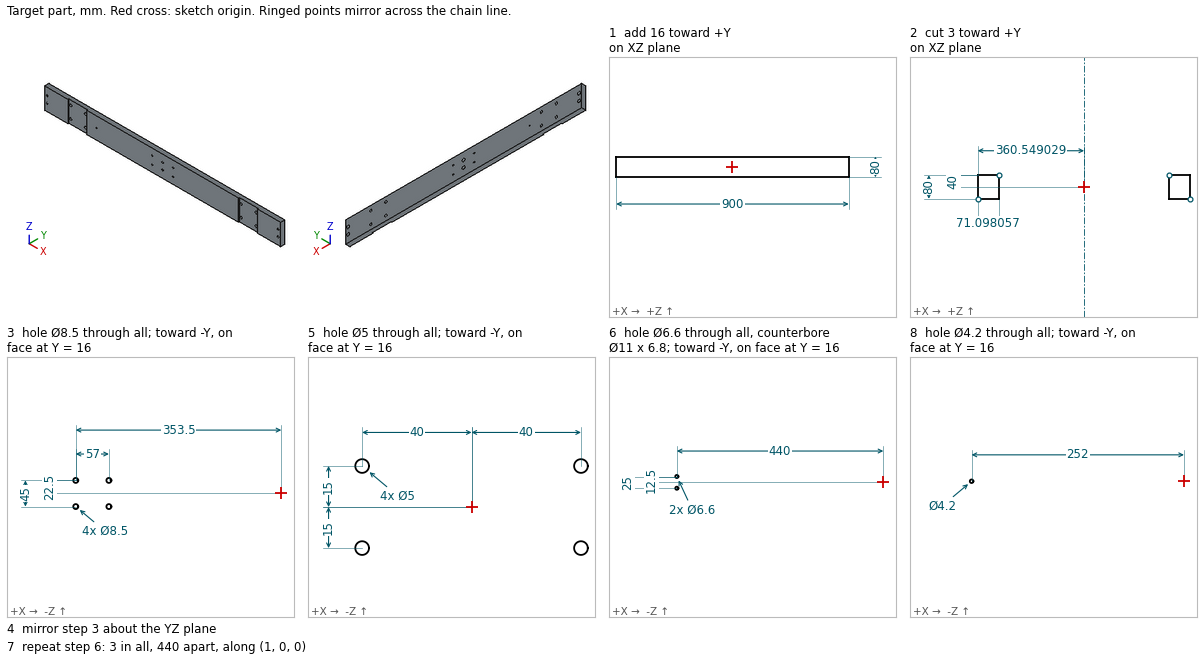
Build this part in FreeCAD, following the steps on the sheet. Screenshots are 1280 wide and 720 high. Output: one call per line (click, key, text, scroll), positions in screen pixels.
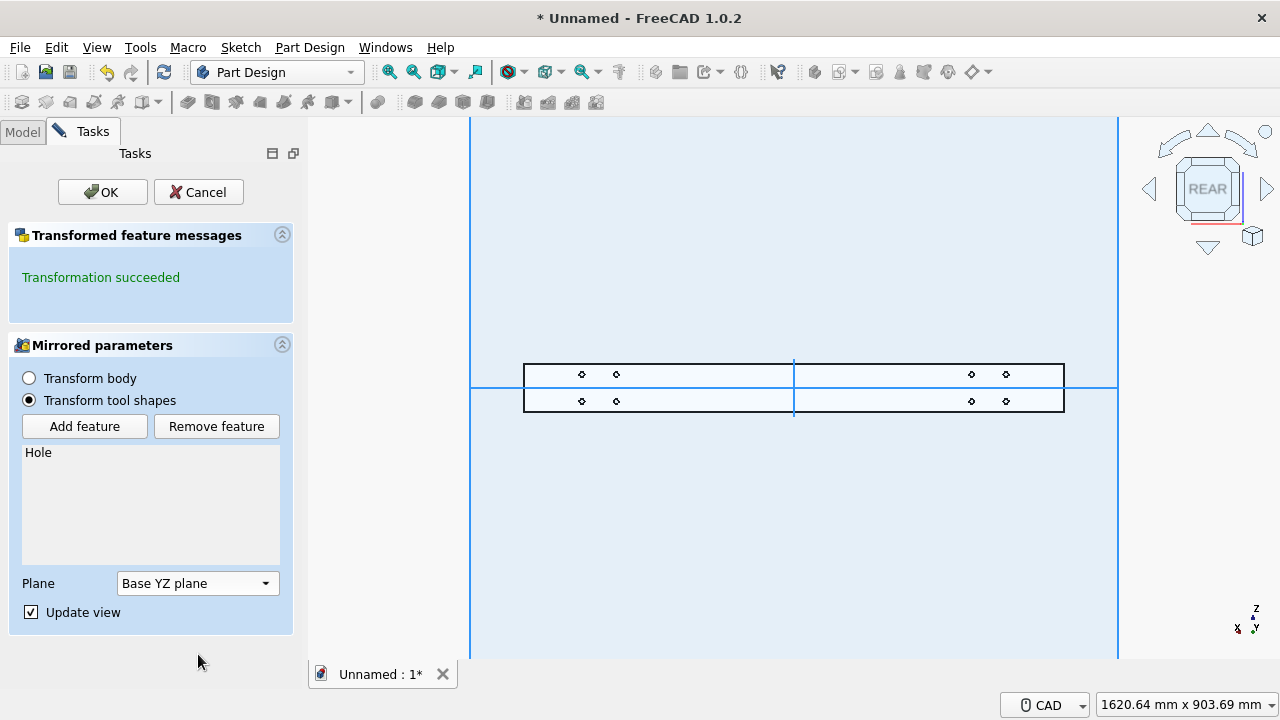
click(103, 192)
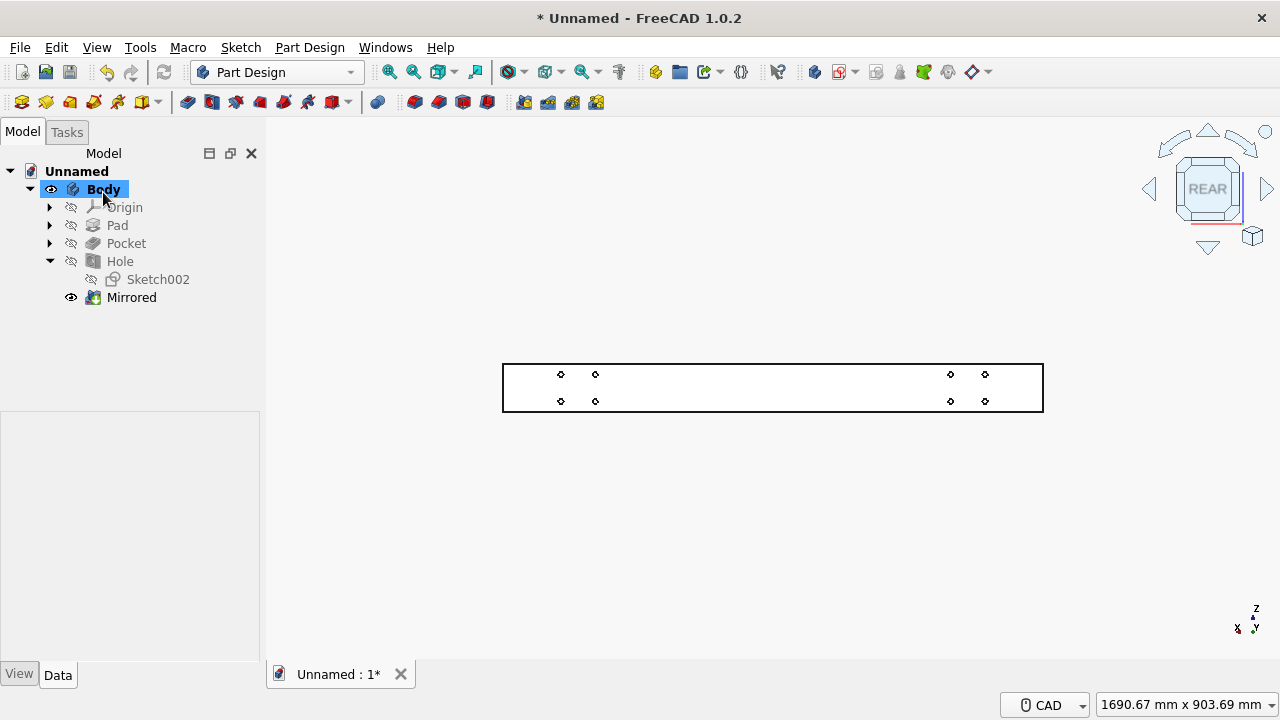
click(619, 387)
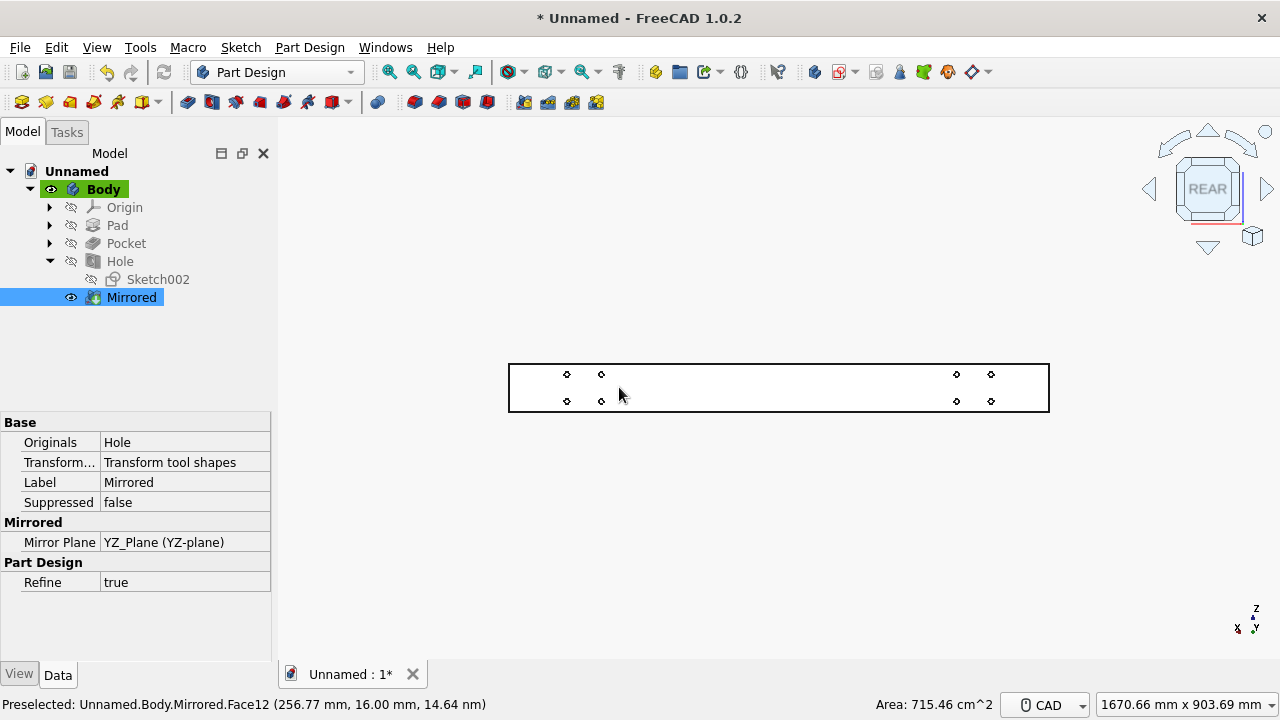
click(840, 72)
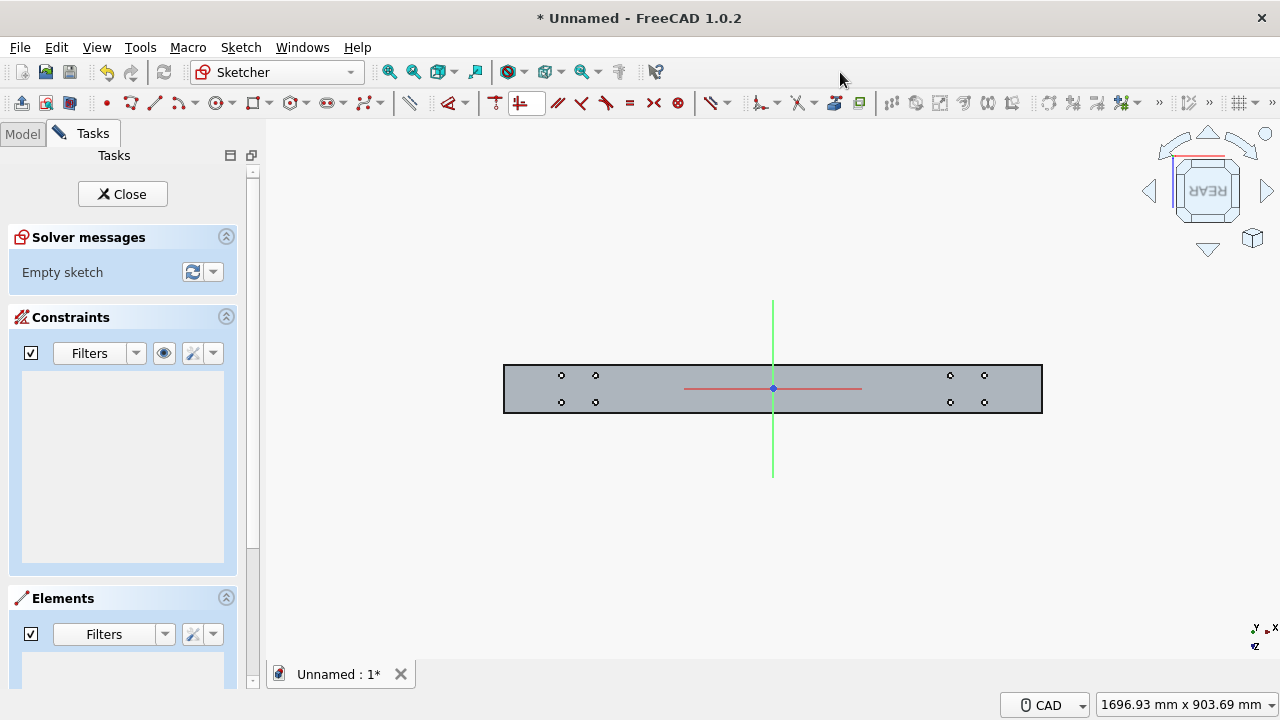
scroll(780, 389, up, 12)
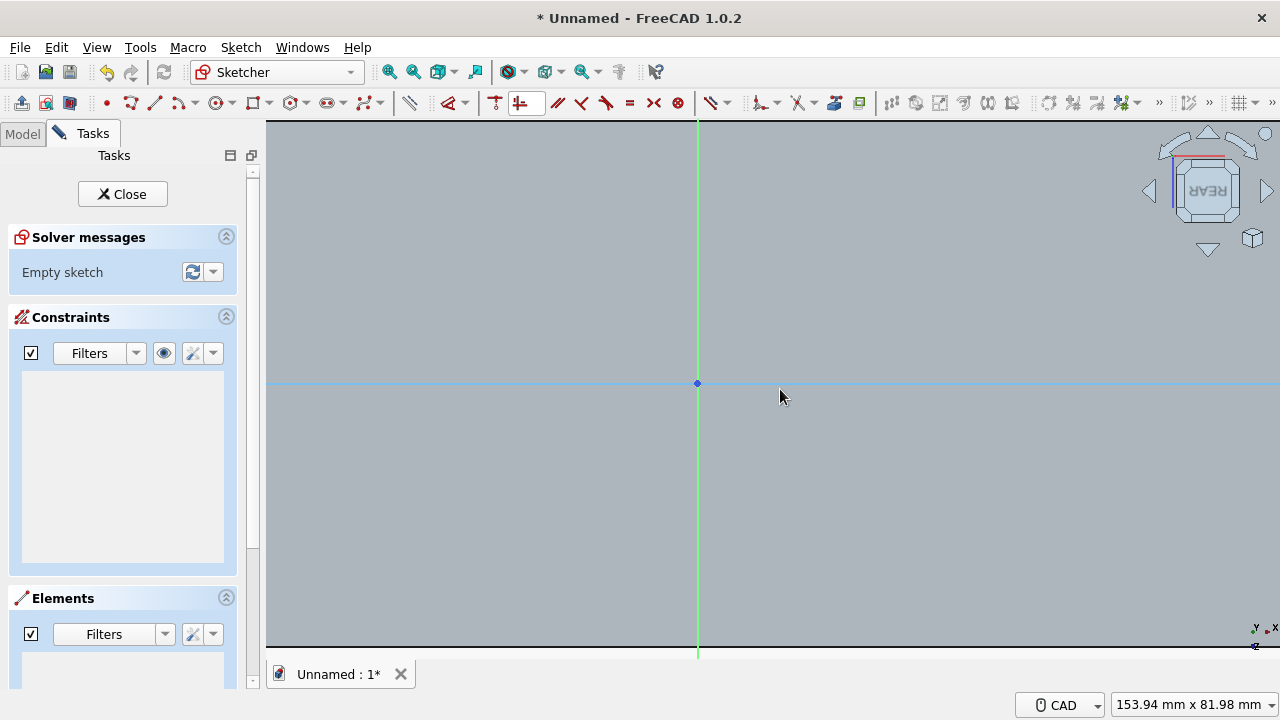
click(216, 104)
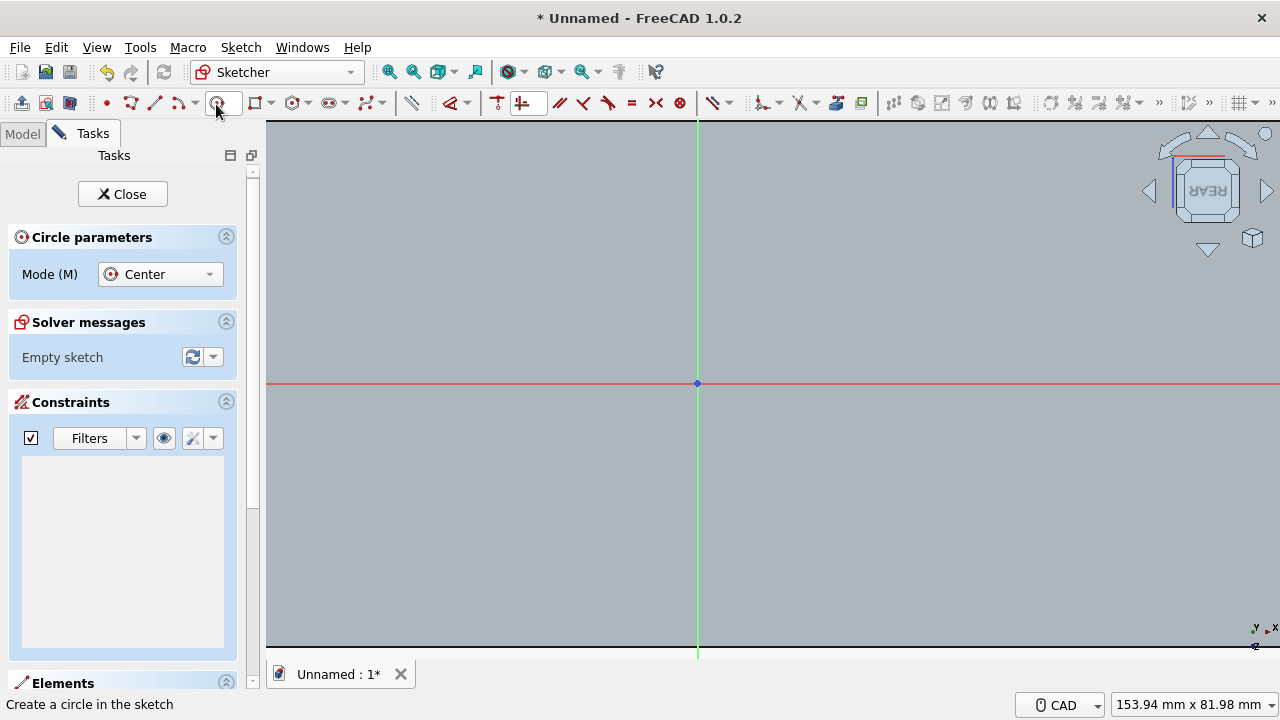
scroll(434, 285, up, 2)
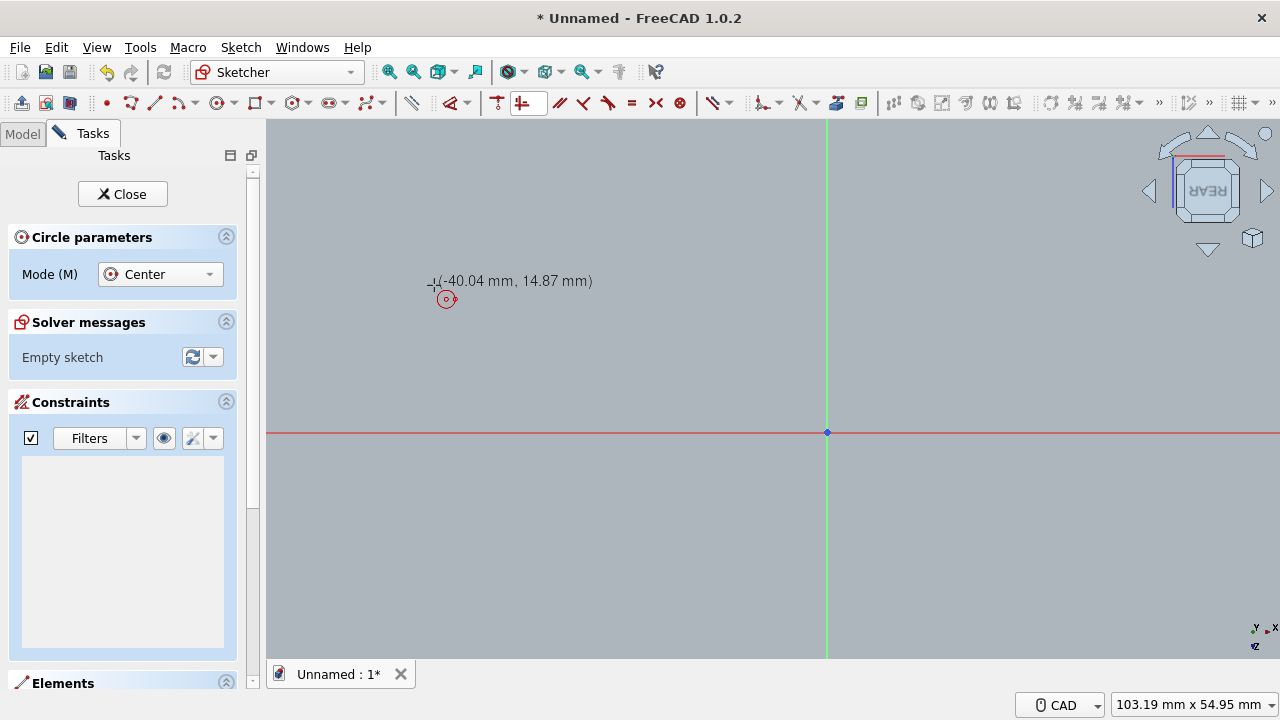
click(434, 285)
click(452, 268)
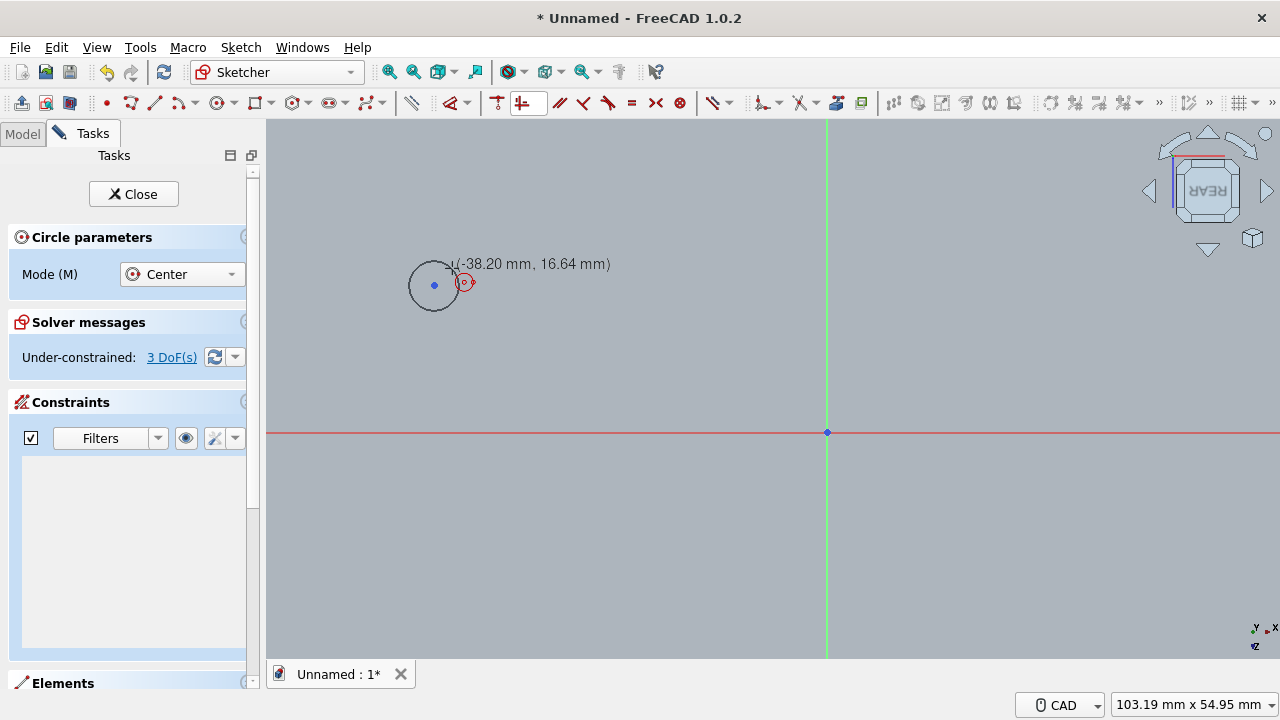
scroll(455, 301, down, 2)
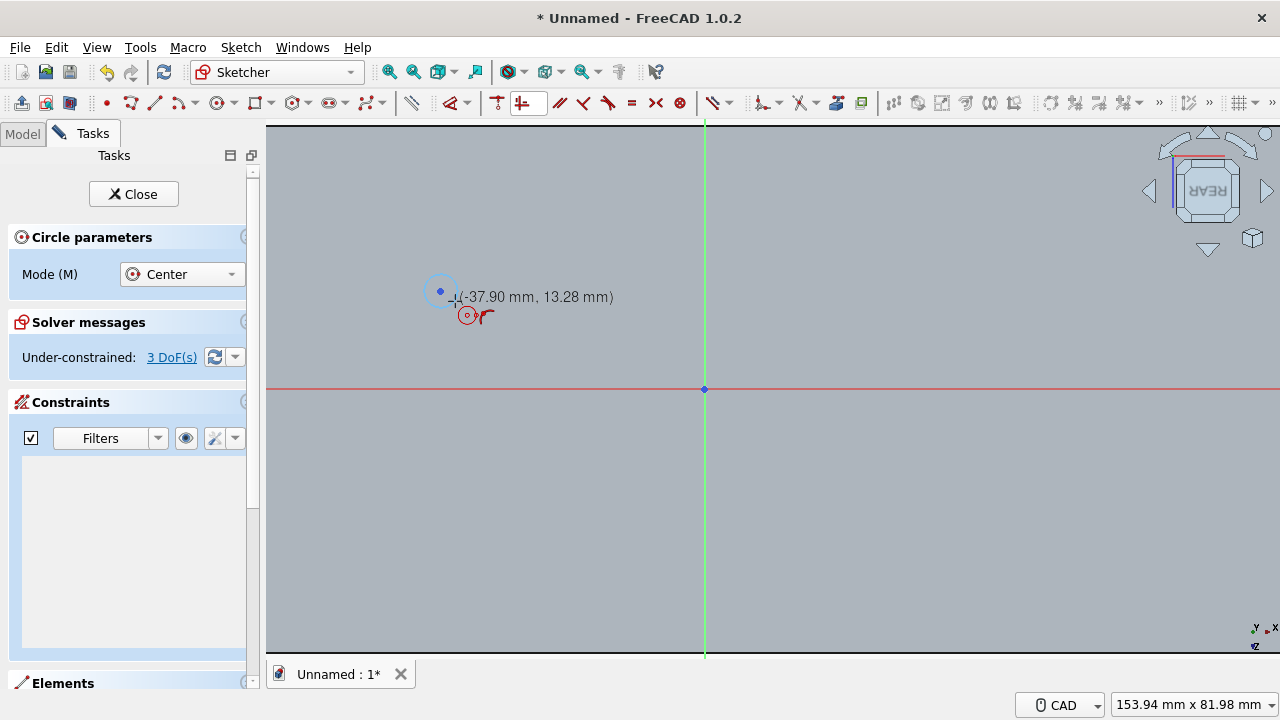
scroll(968, 290, up, 2)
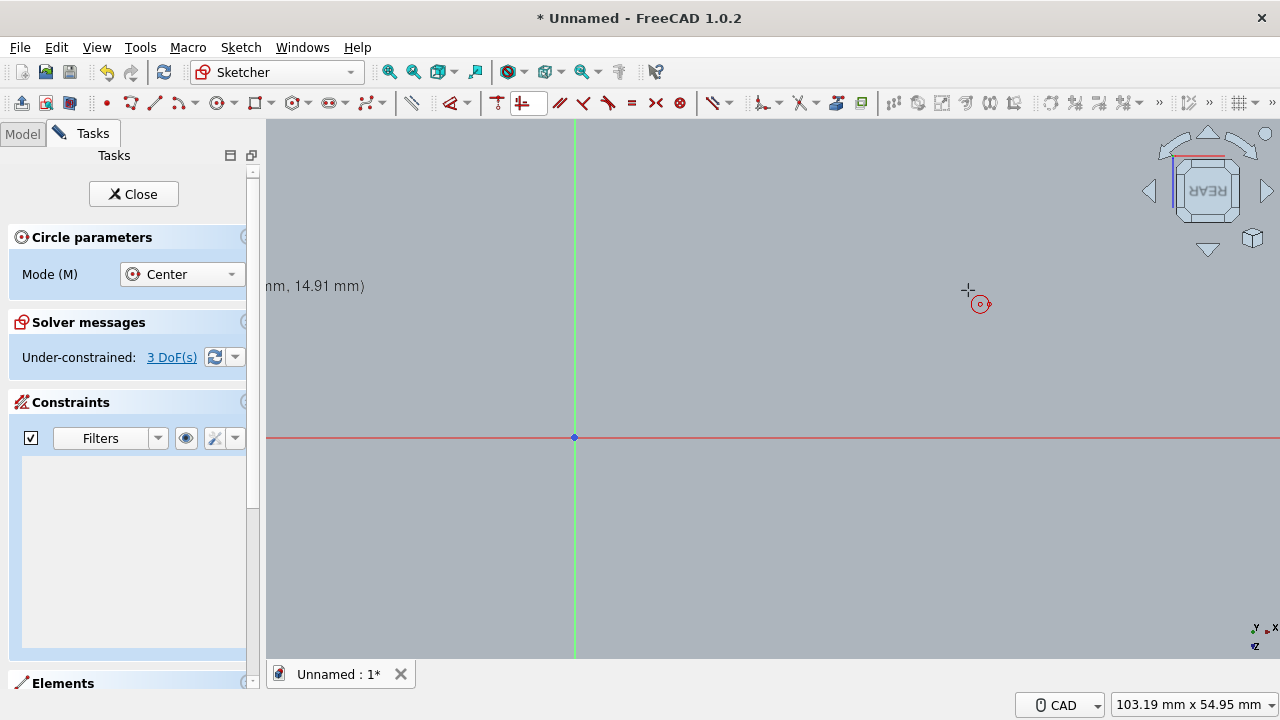
click(968, 291)
click(985, 273)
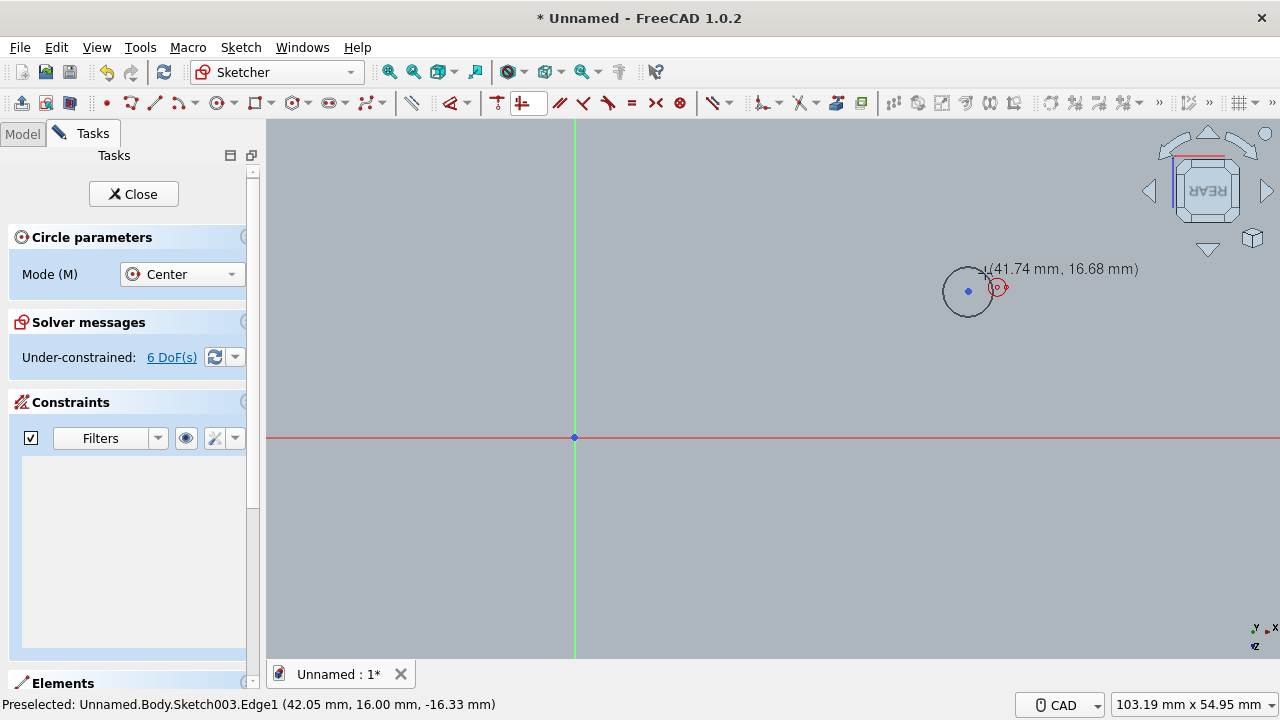
scroll(968, 290, down, 2)